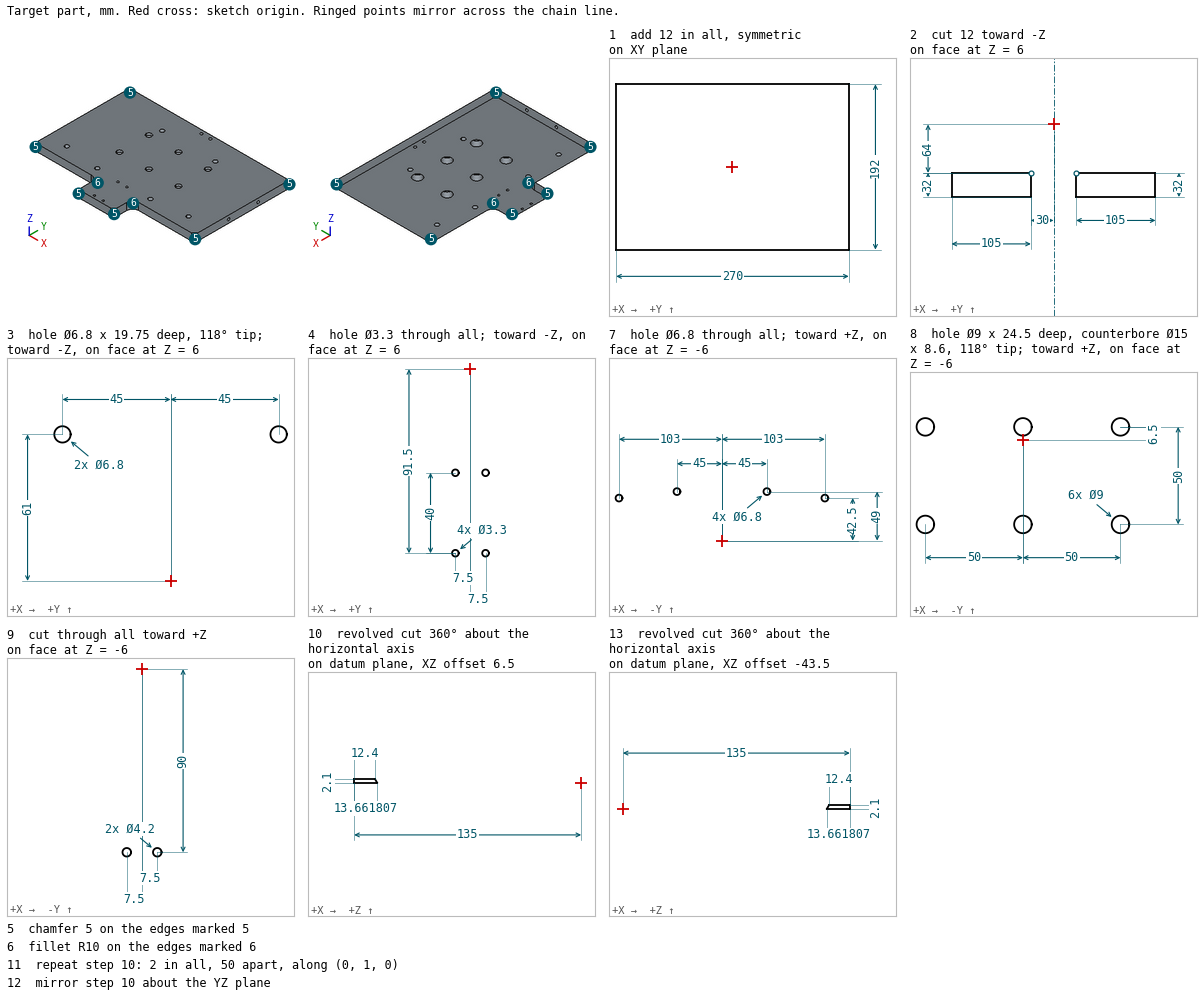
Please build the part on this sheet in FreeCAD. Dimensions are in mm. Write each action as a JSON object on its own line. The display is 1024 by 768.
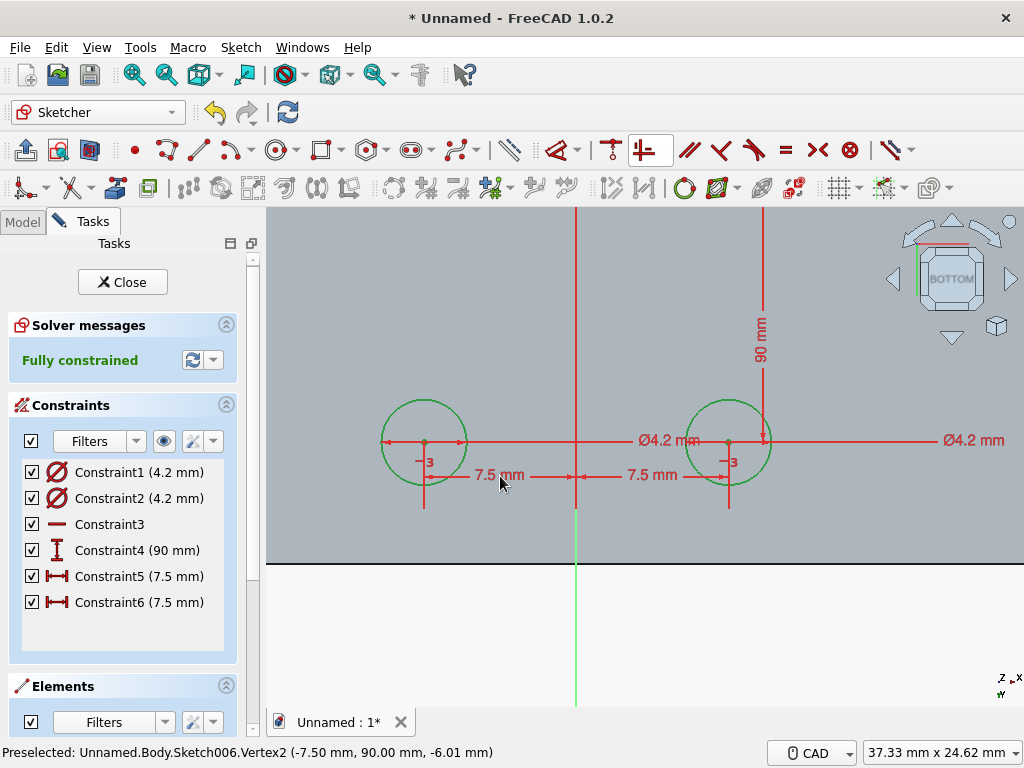
{"action": "left_click", "coordinate": [123, 282]}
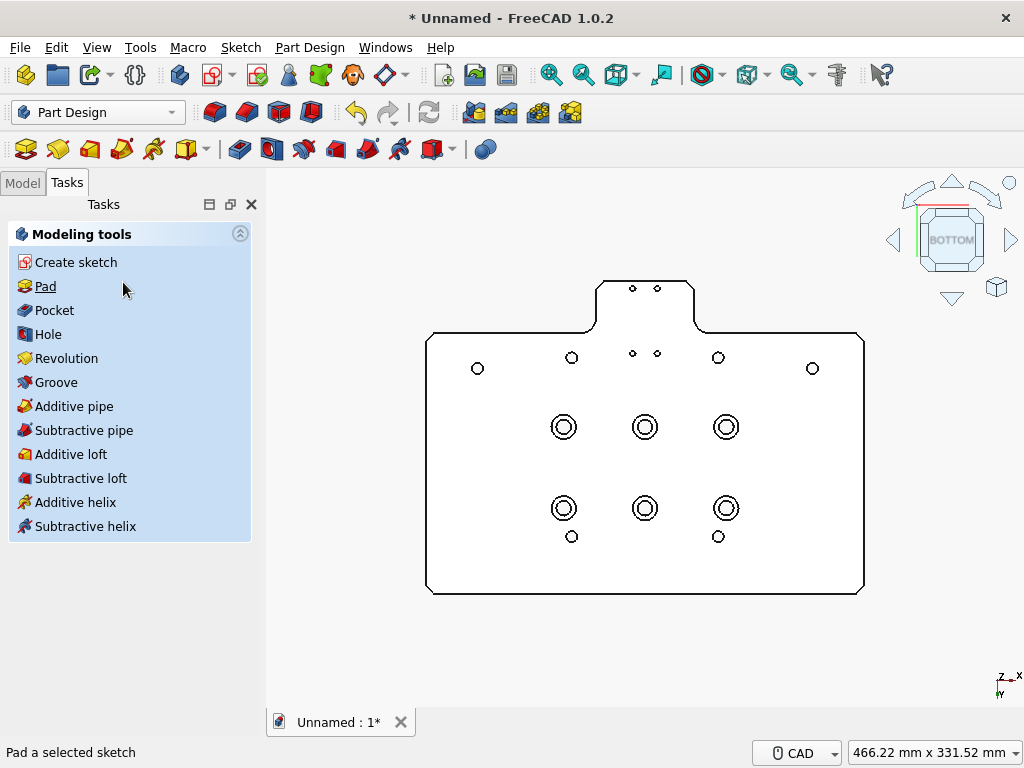
{"action": "left_click", "coordinate": [240, 150]}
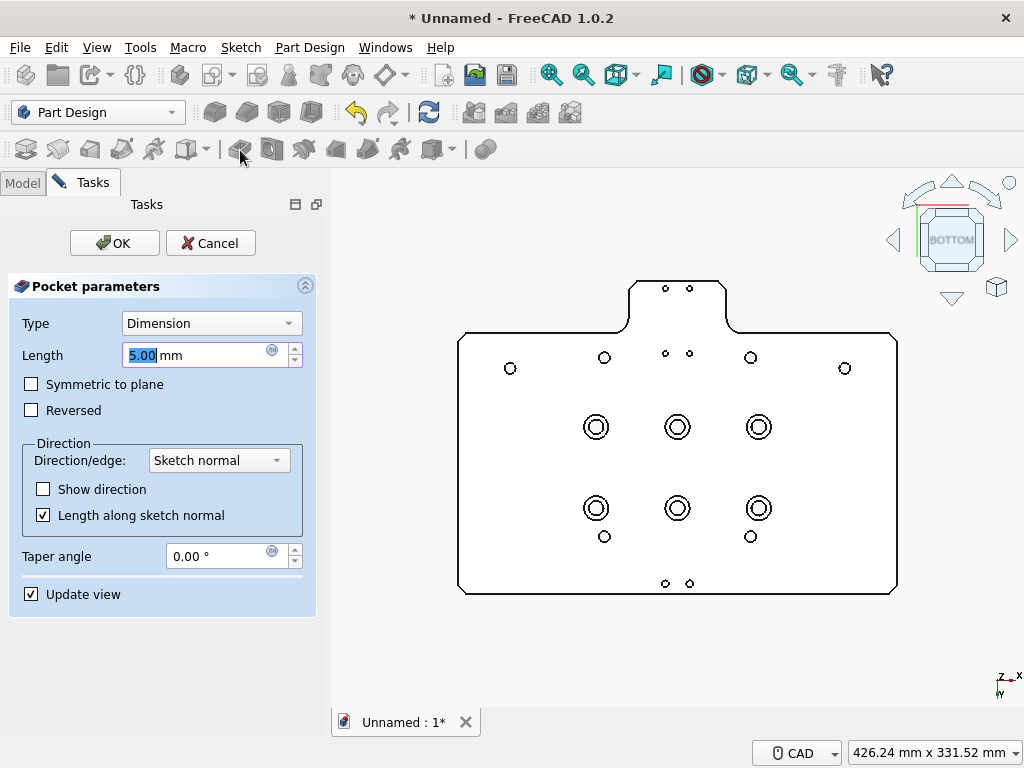
{"action": "left_click", "coordinate": [212, 324]}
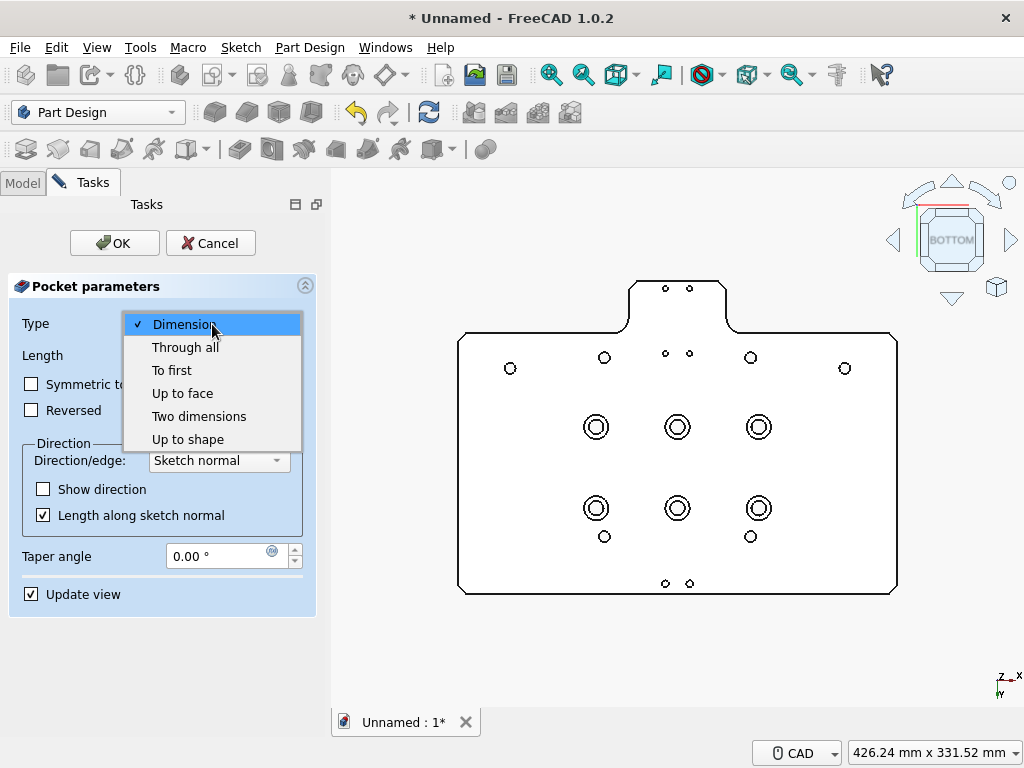
{"action": "left_click", "coordinate": [212, 348]}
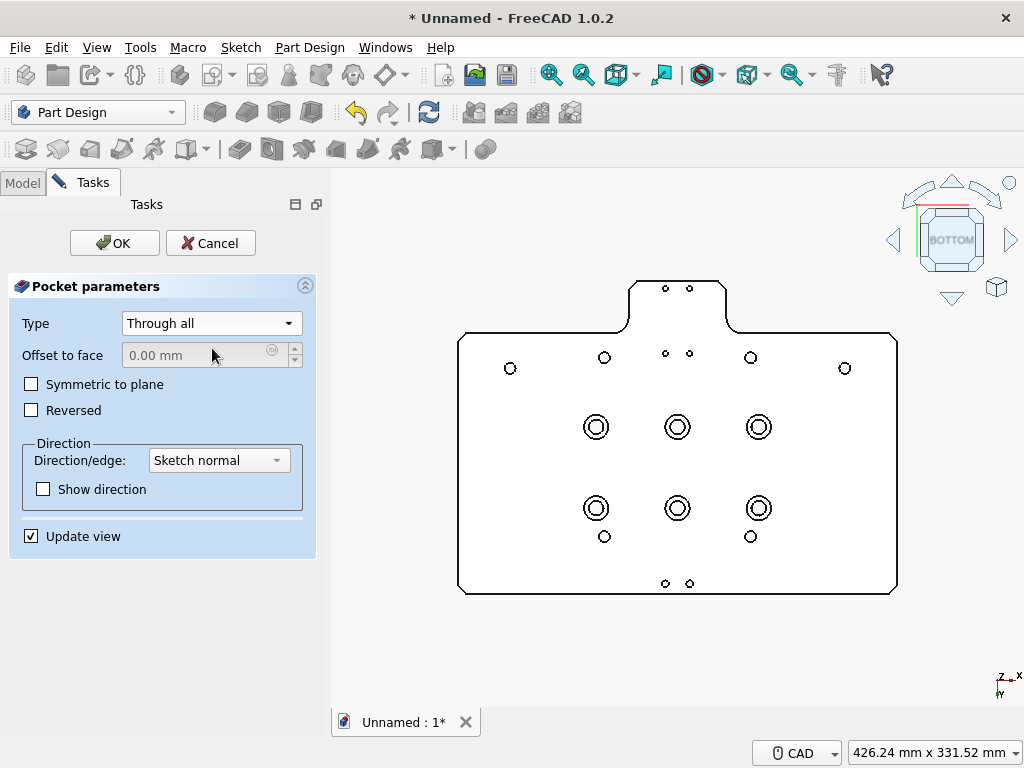
{"action": "left_click", "coordinate": [115, 243]}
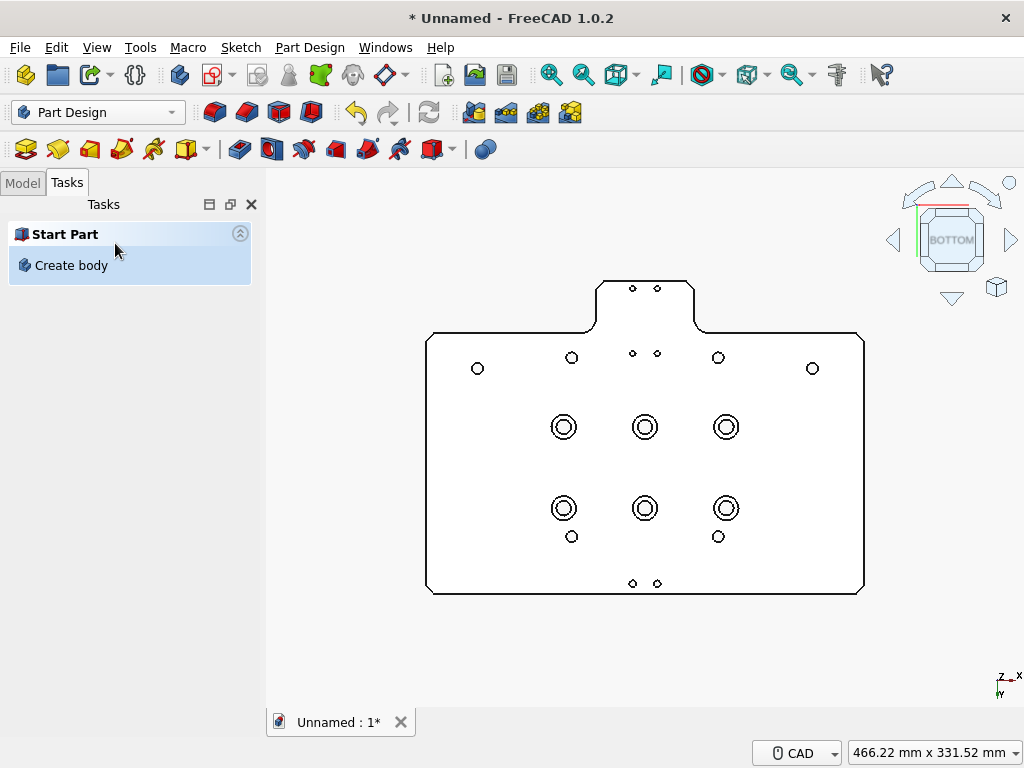
{"action": "left_click", "coordinate": [23, 182]}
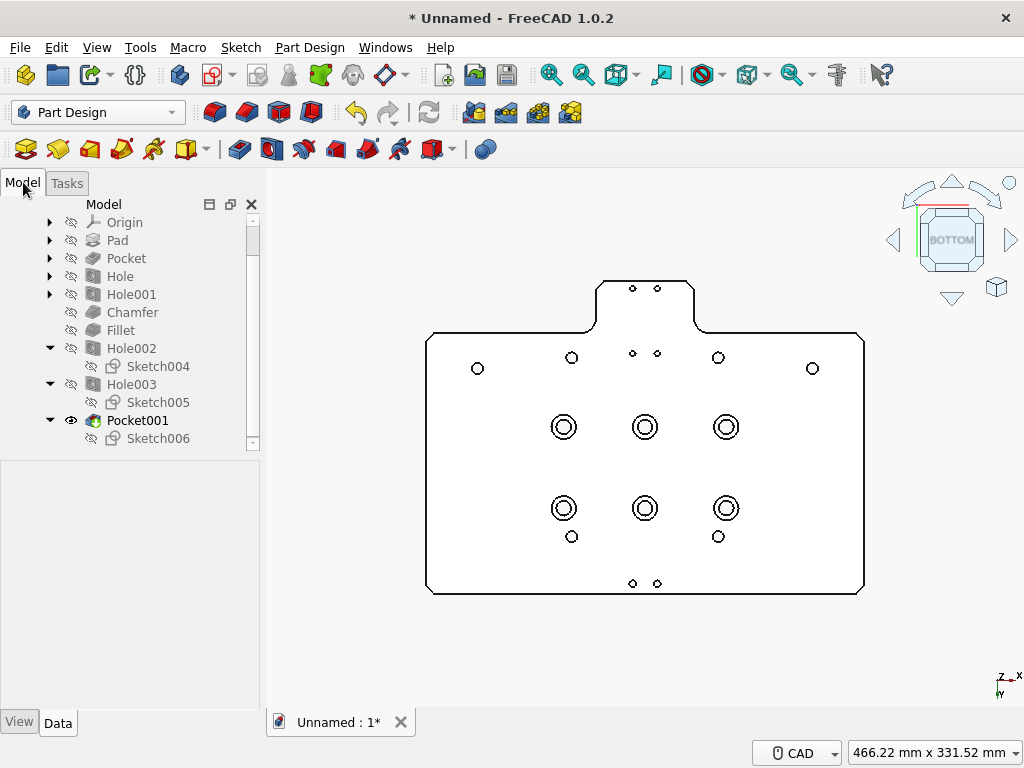
{"action": "left_click", "coordinate": [50, 222]}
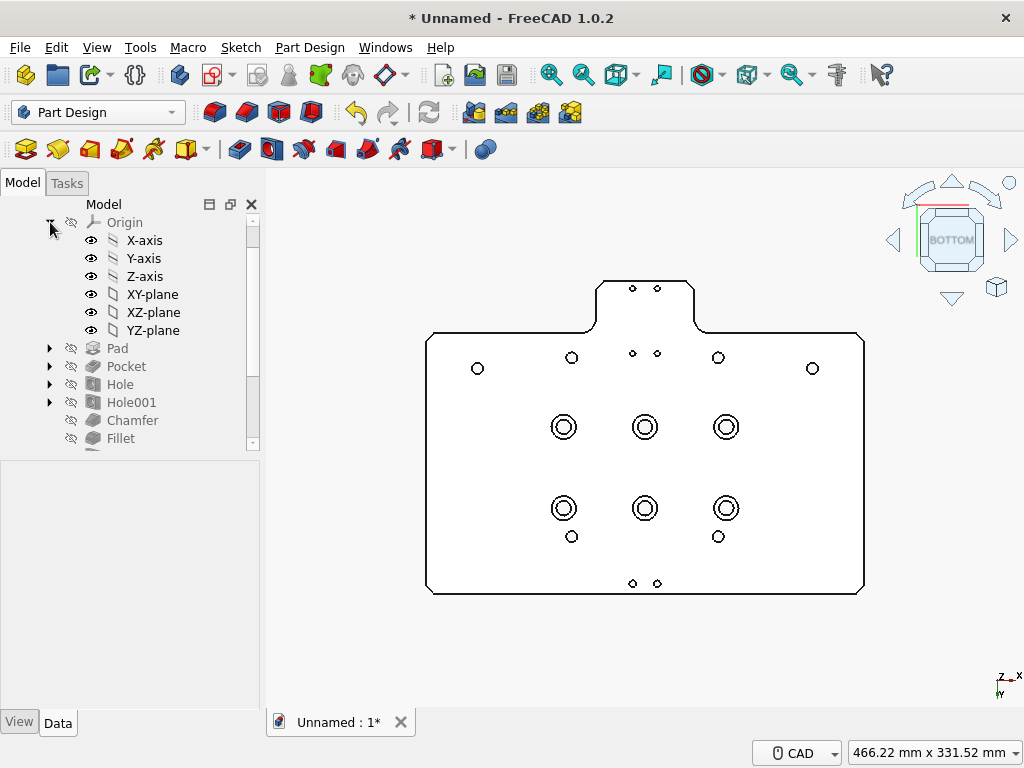
{"action": "left_click", "coordinate": [136, 312]}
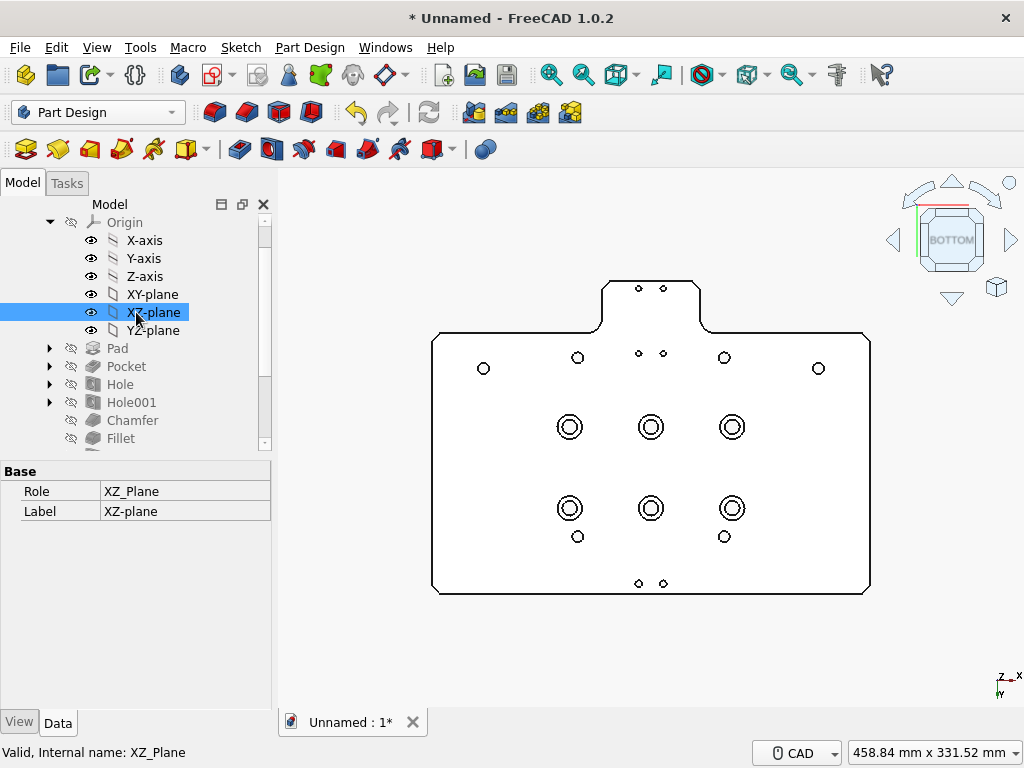
{"action": "left_click", "coordinate": [386, 76]}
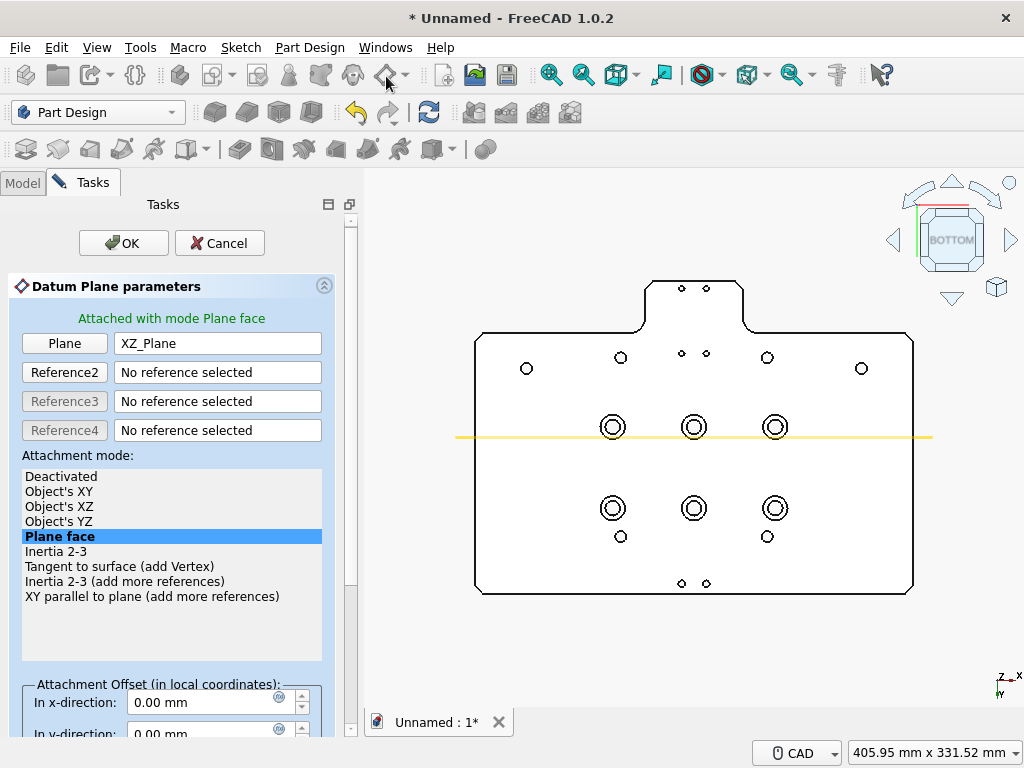
{"action": "scroll", "coordinate": [351, 475], "scroll_direction": "down", "scroll_amount": 2}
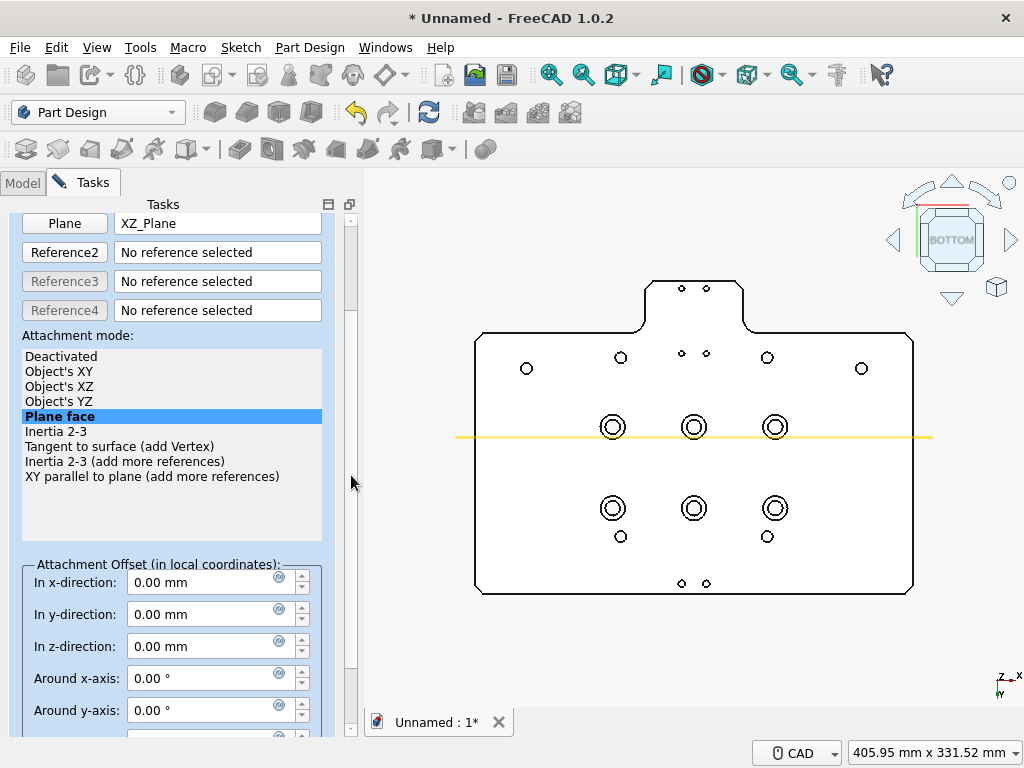
{"action": "triple_click", "coordinate": [210, 646]}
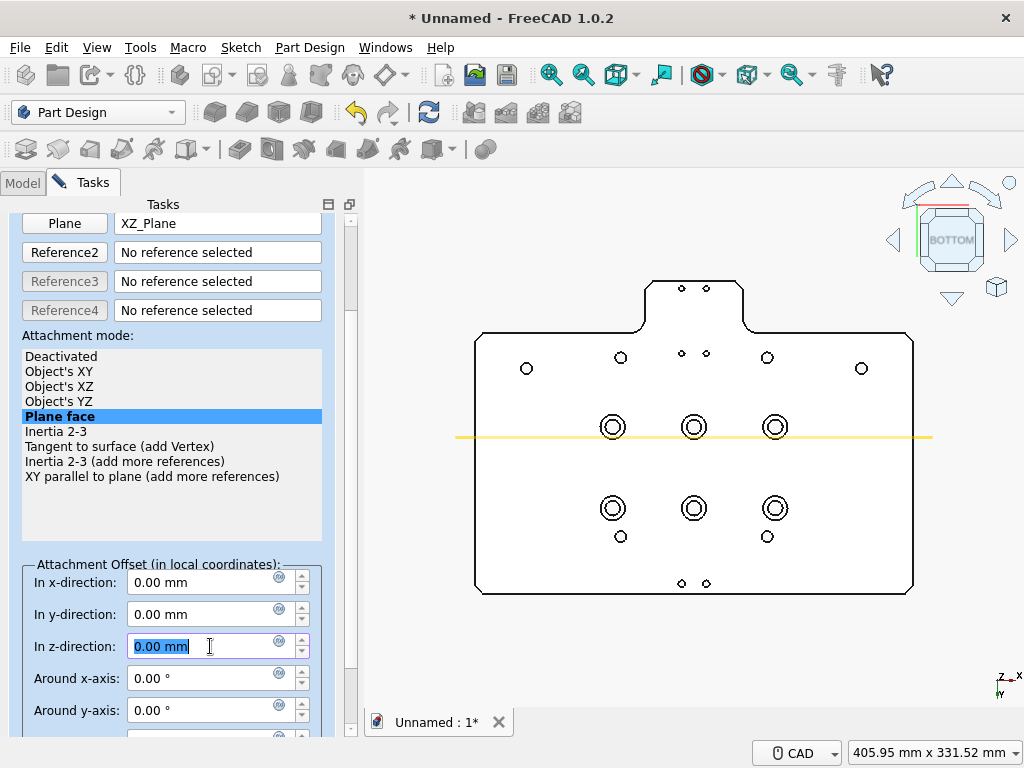
{"action": "type", "text": "6.5"}
{"action": "key", "text": "Tab"}